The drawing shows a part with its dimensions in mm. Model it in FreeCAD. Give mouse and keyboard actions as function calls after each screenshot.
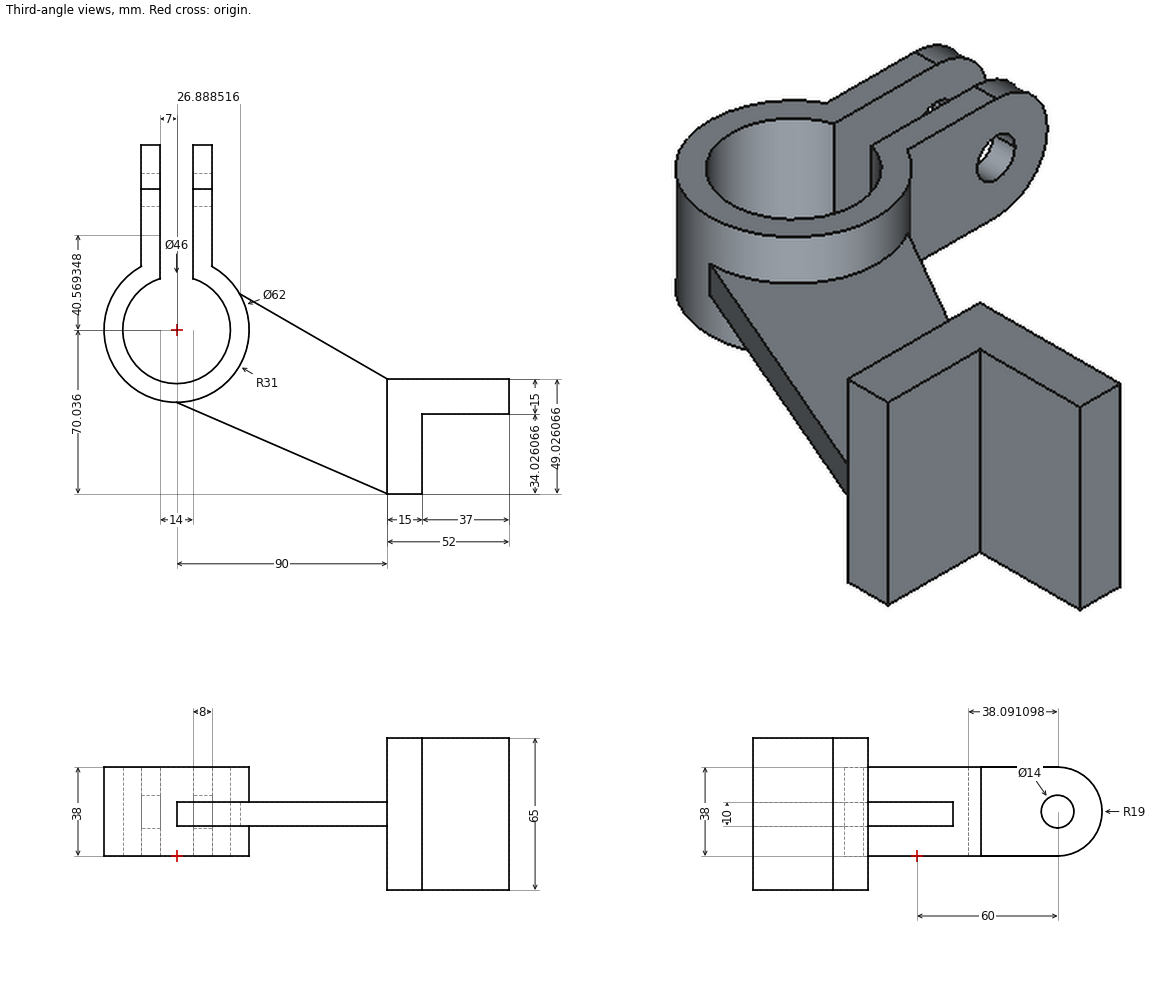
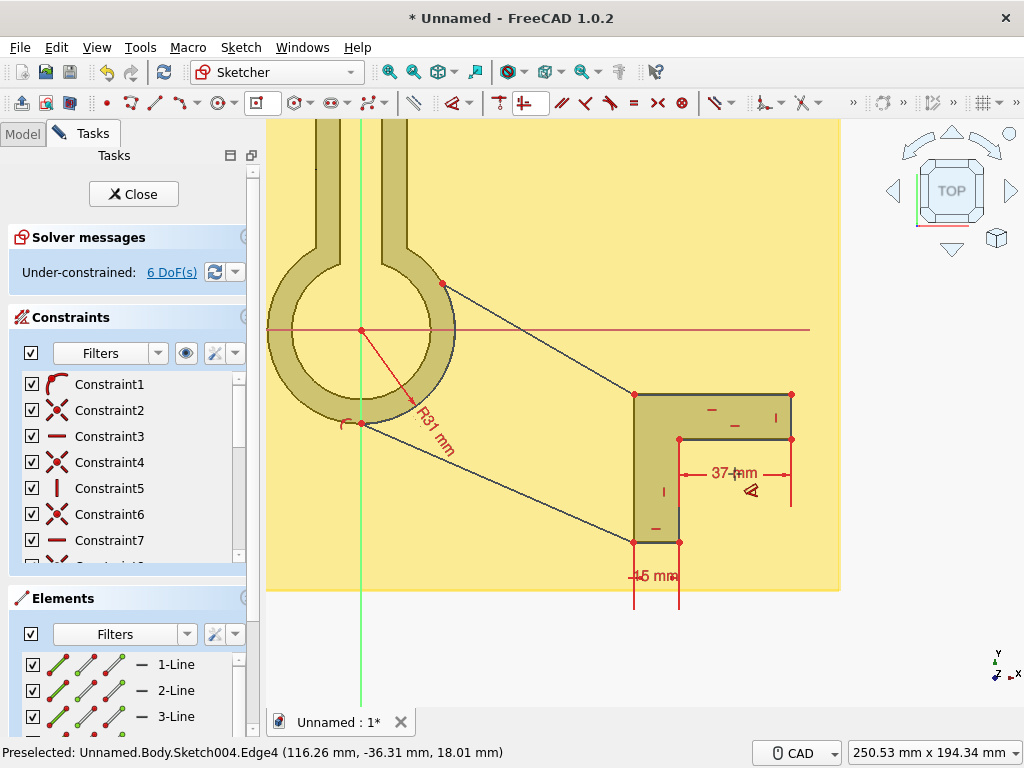
click(791, 427)
click(825, 418)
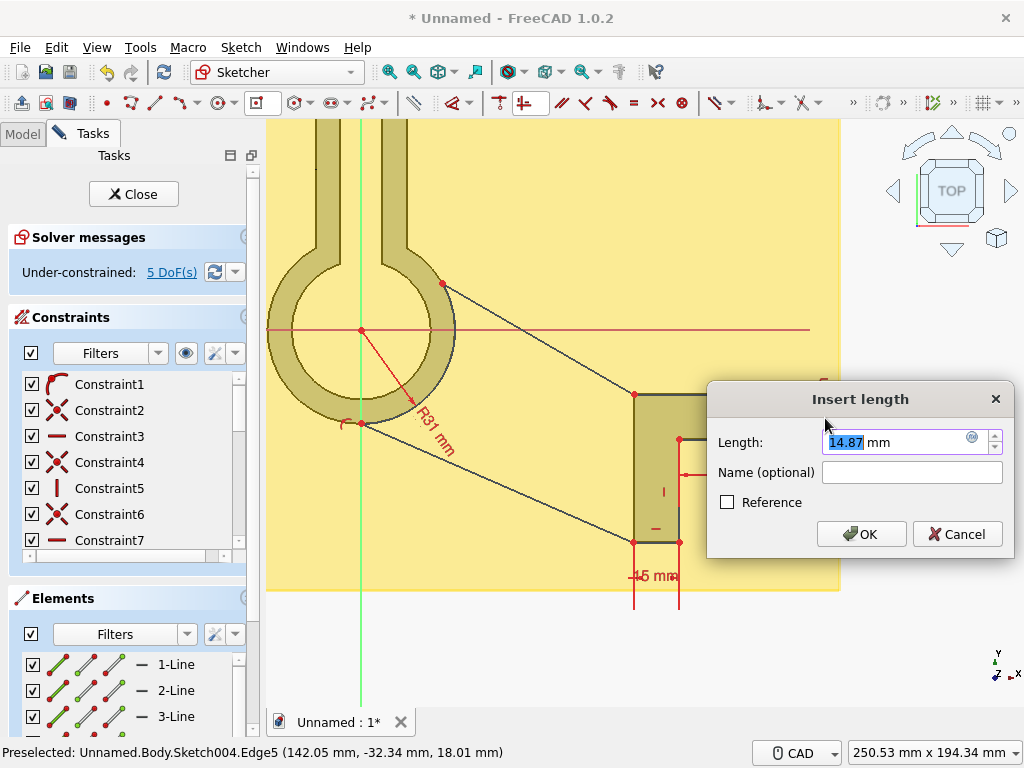
text(15)
key(Return)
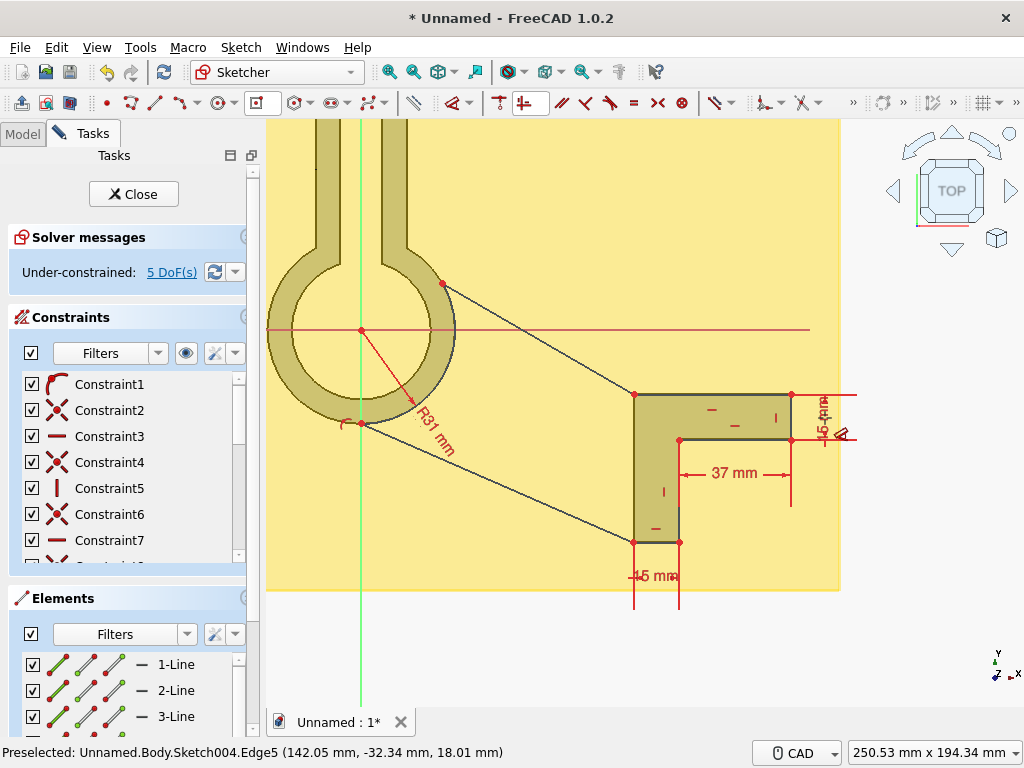
click(744, 395)
click(713, 361)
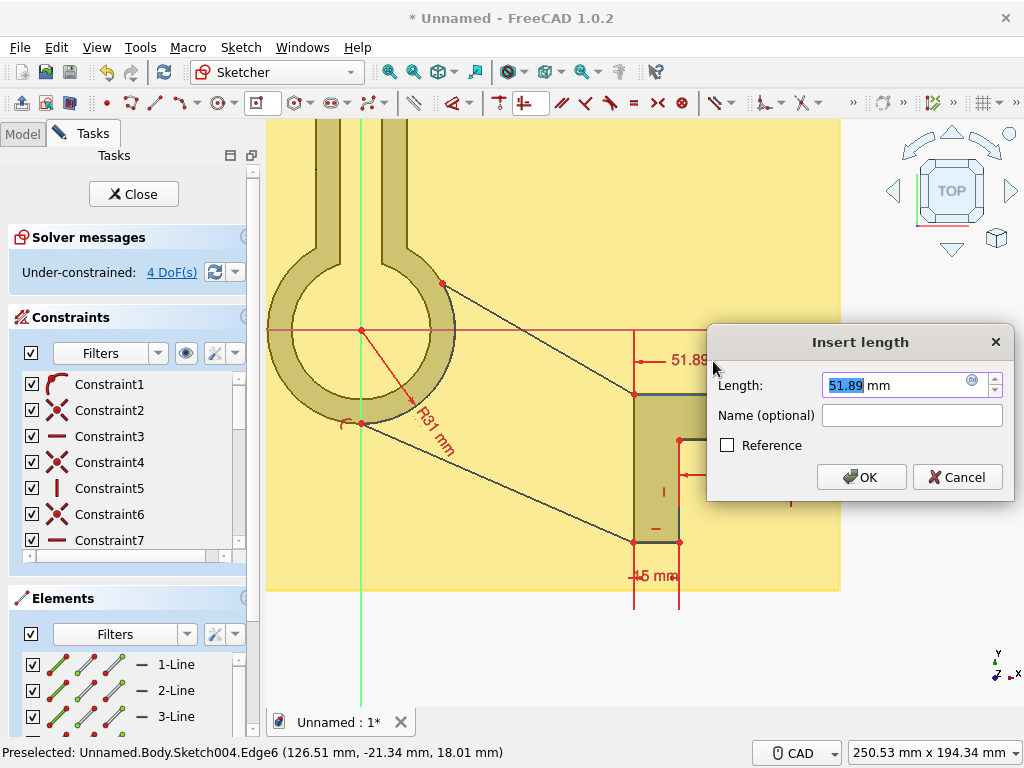
text(52)
key(Return)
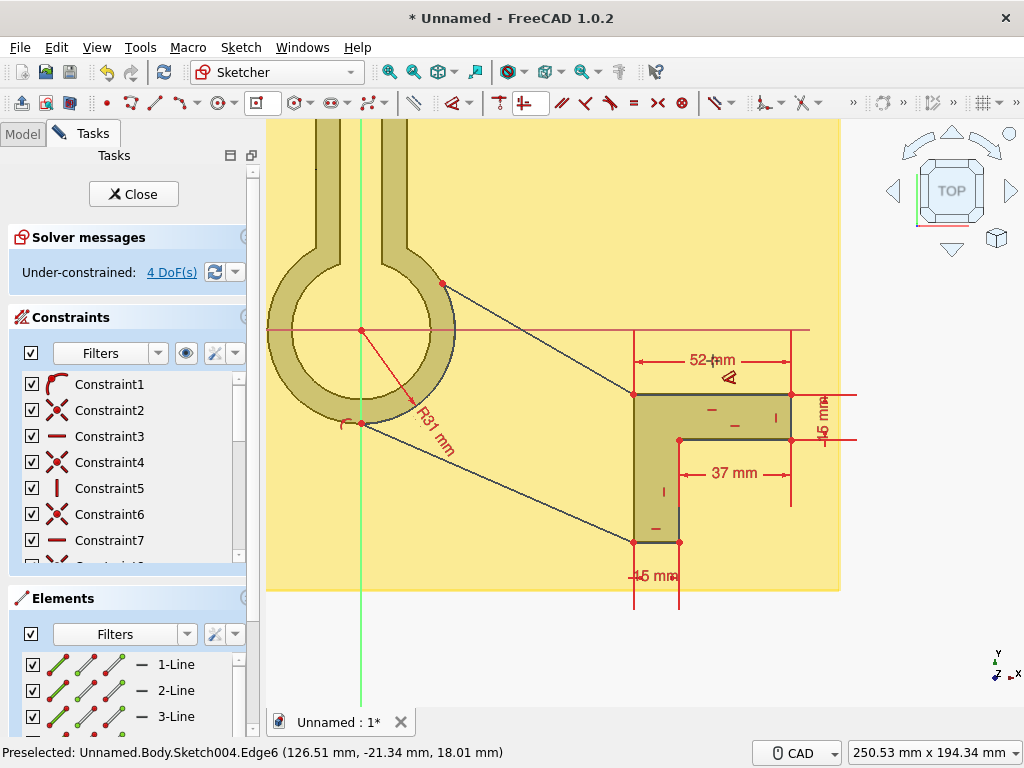
click(634, 543)
click(497, 577)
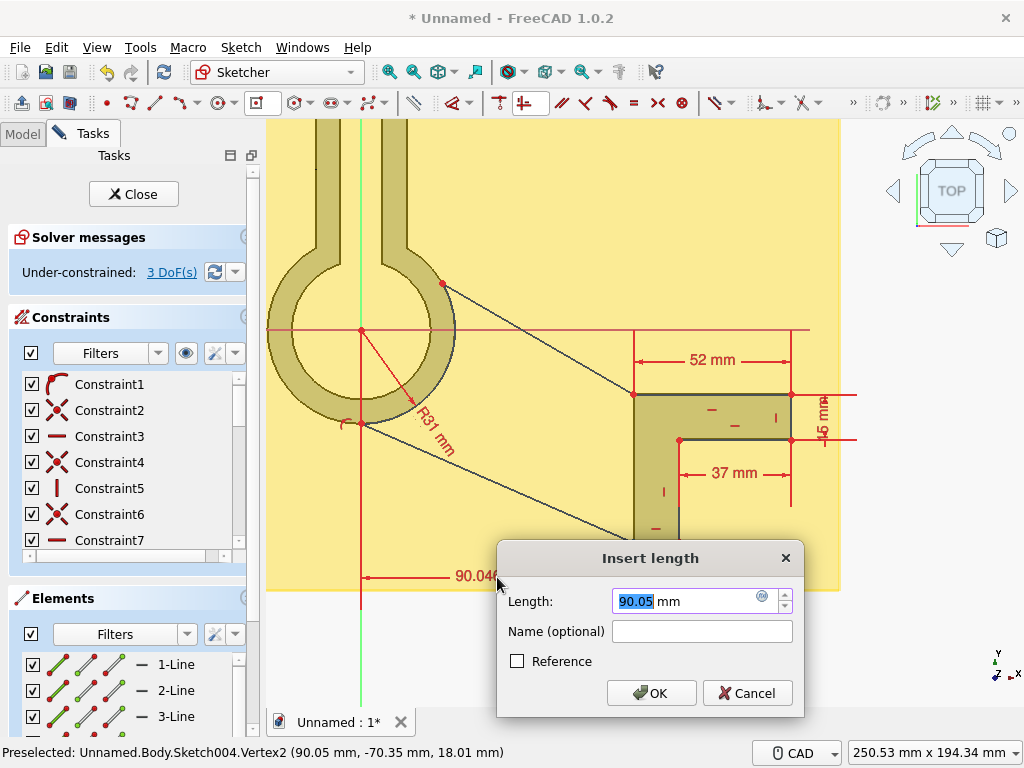
text(90)
key(Return)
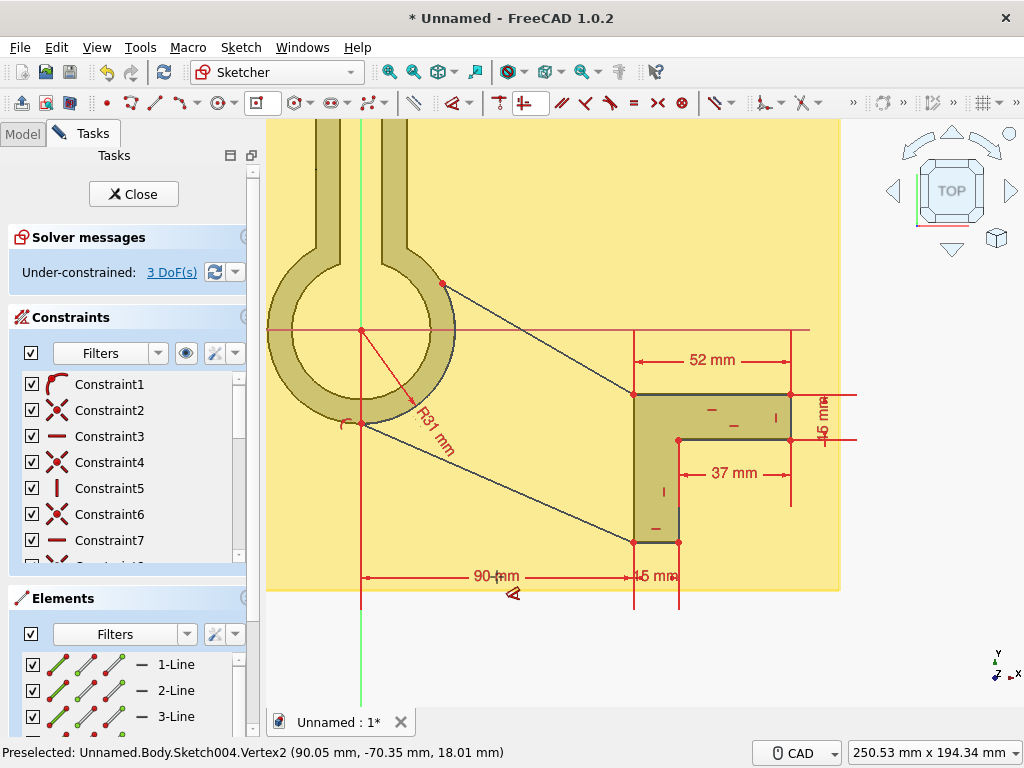
click(634, 543)
click(327, 437)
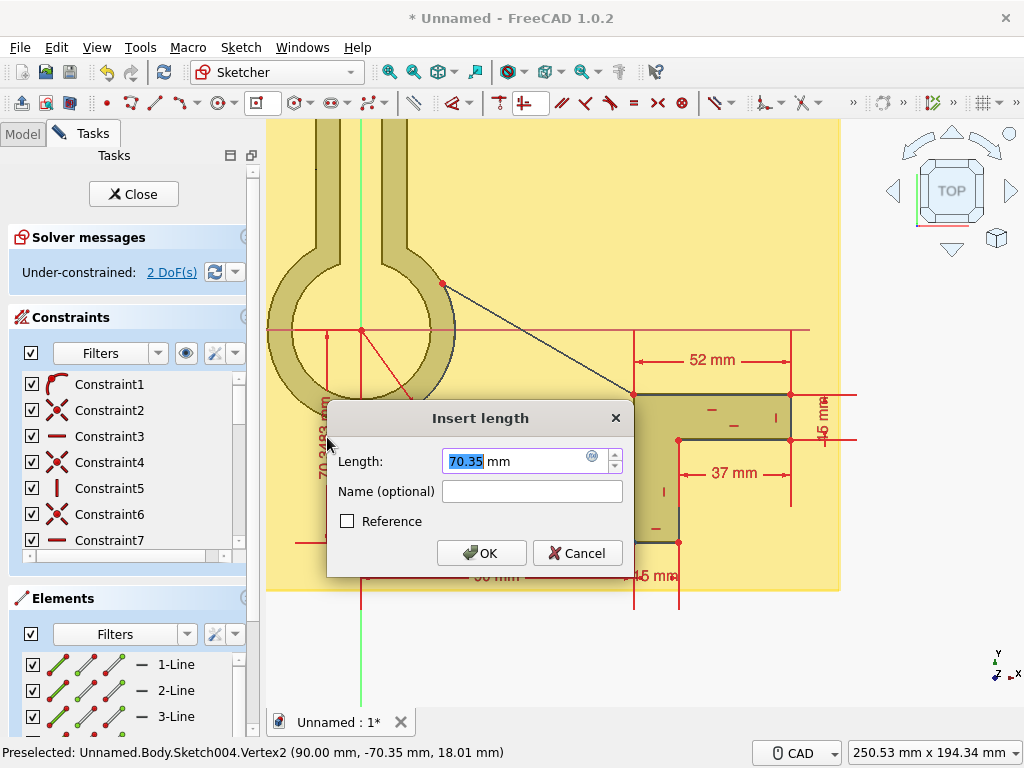
text(70.036)
key(Return)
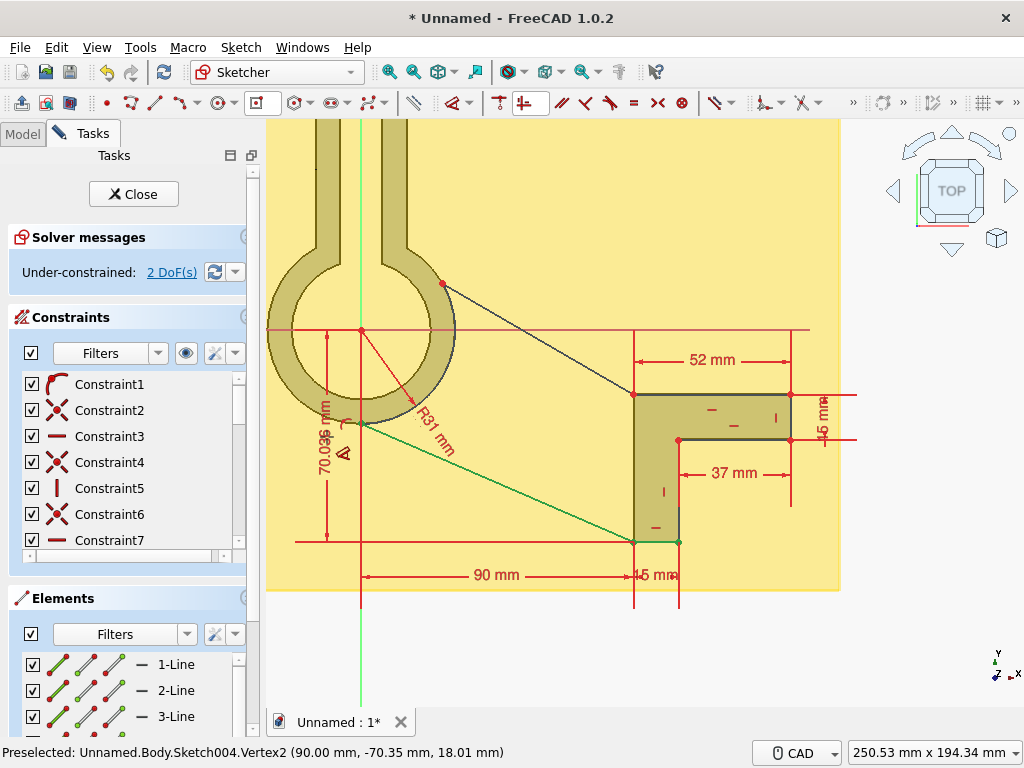
click(679, 511)
click(713, 515)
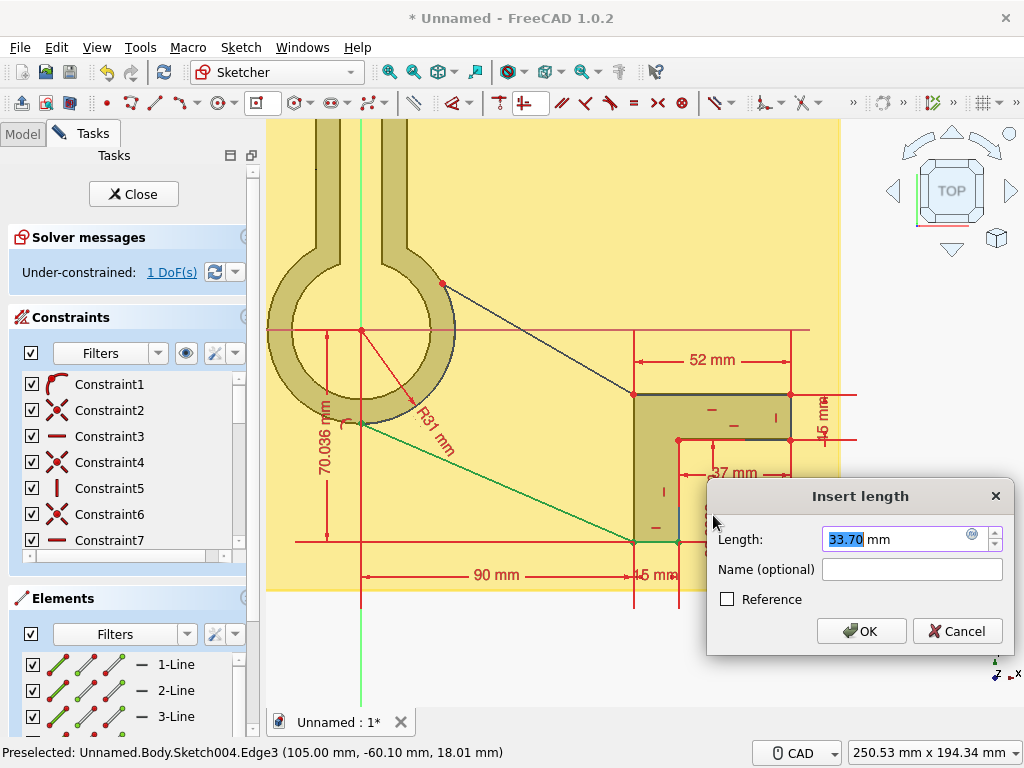
text(34.026066)
key(Return)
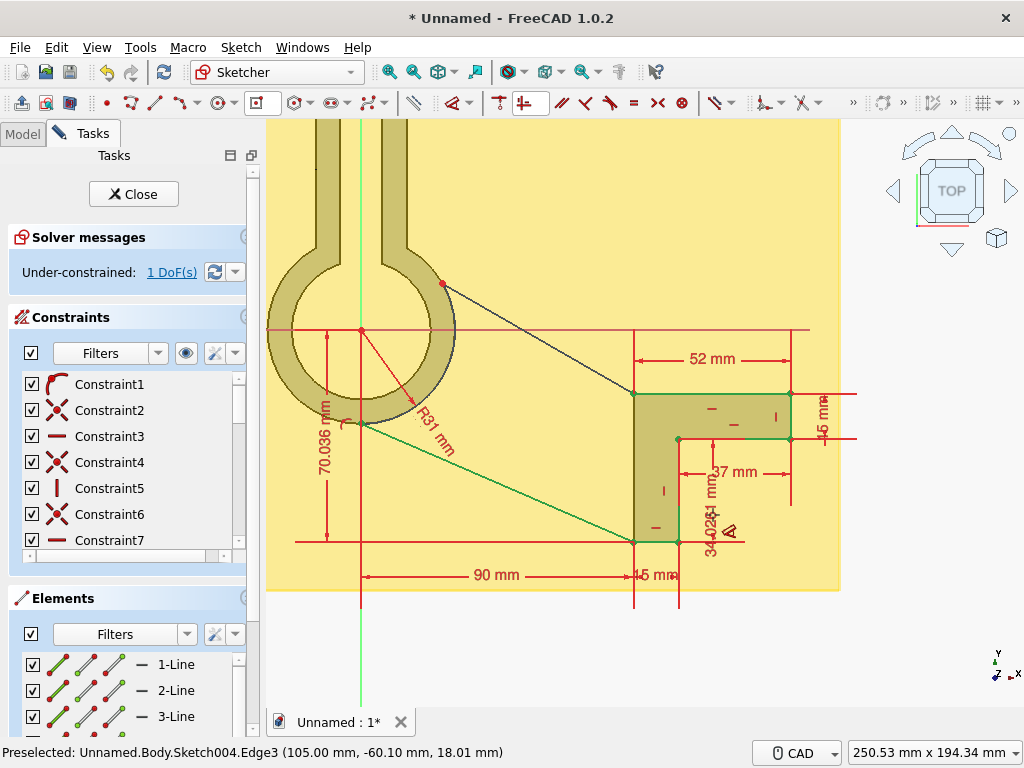
click(443, 284)
click(402, 250)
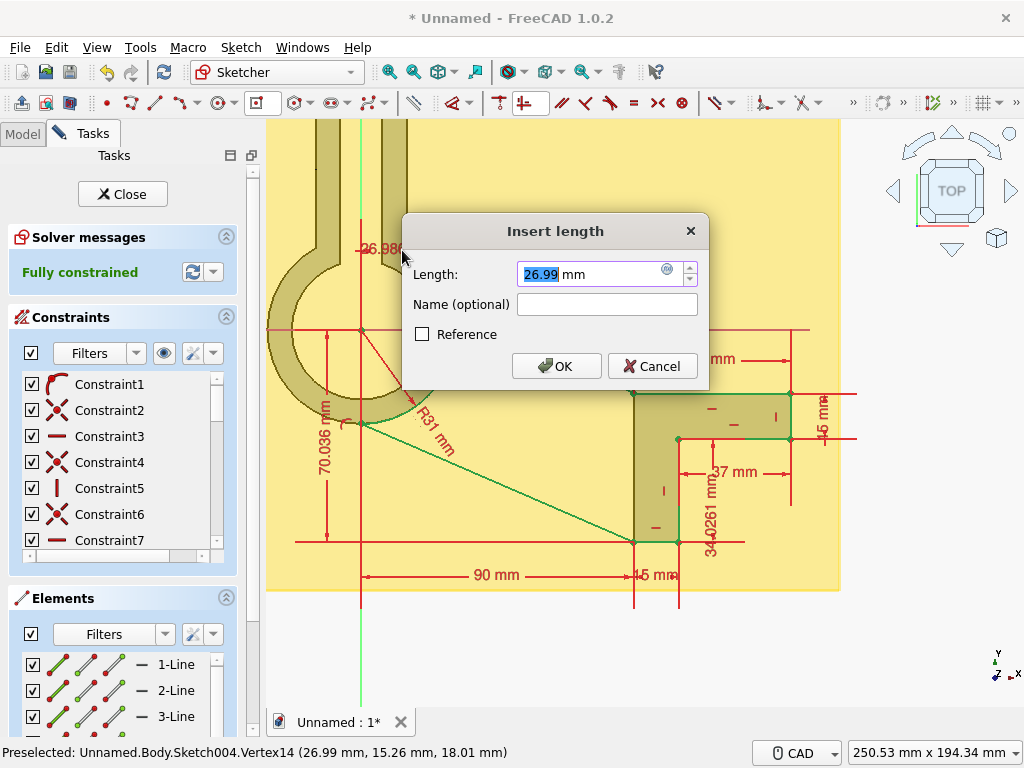
text(26.888516)
key(Return)
key(Escape)